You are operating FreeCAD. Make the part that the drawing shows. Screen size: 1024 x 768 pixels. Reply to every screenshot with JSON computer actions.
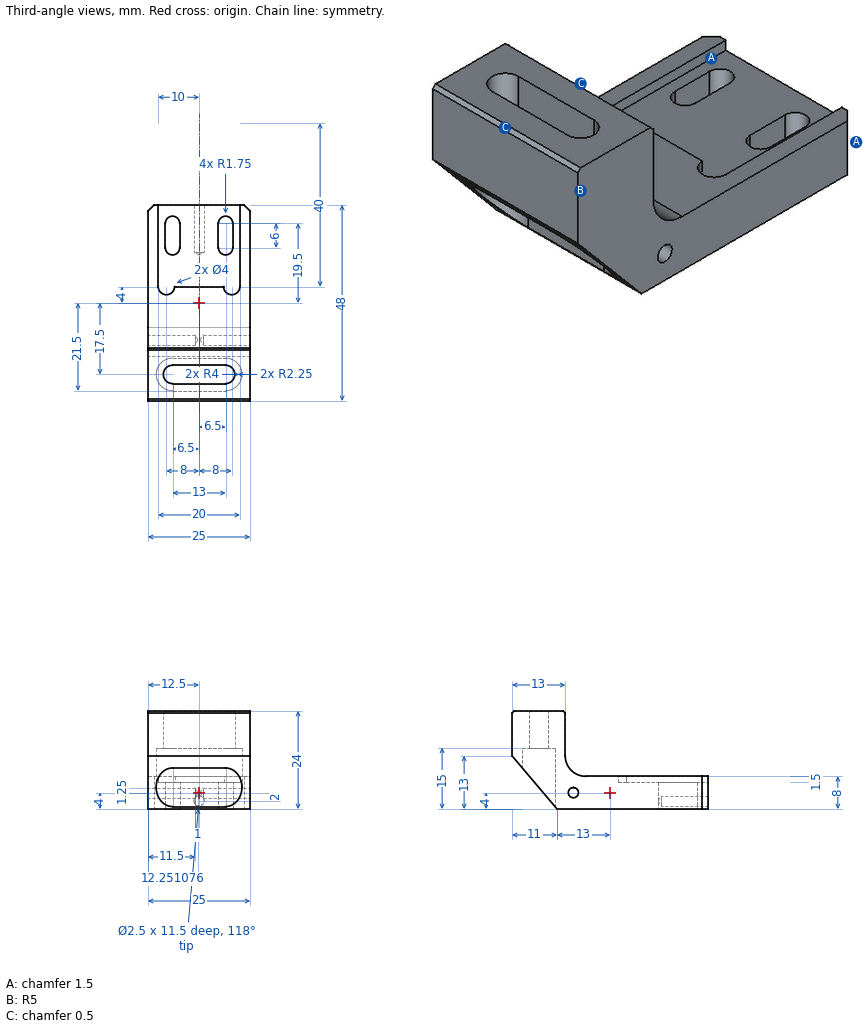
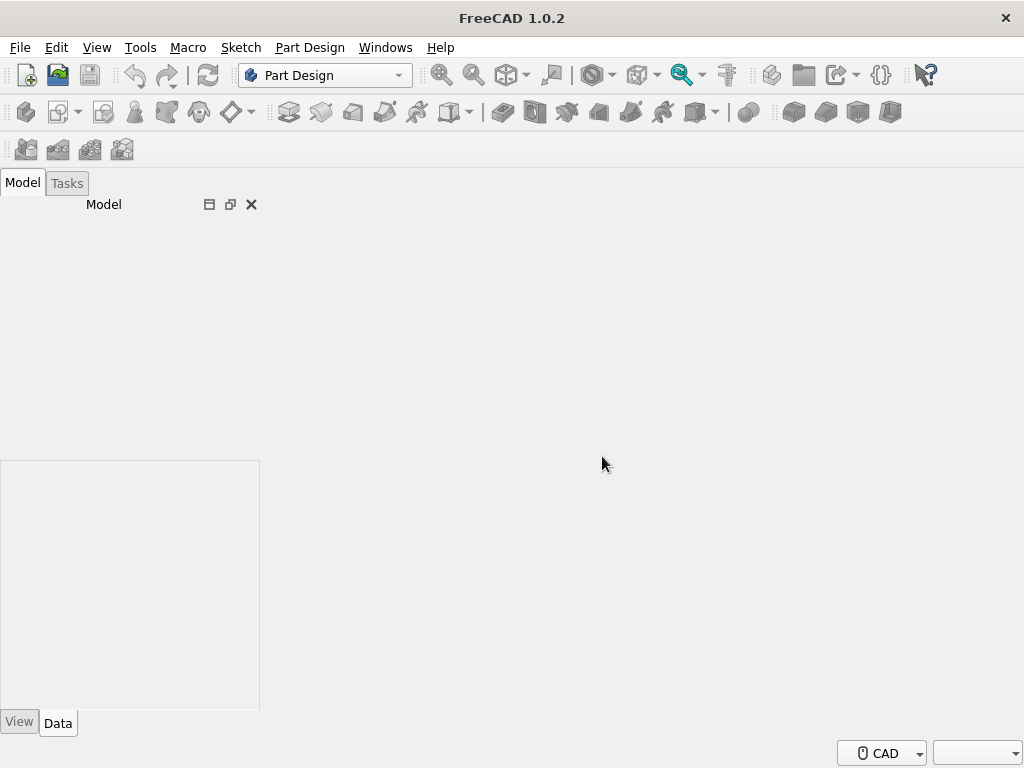
{"action": "left_click", "coordinate": [26, 76]}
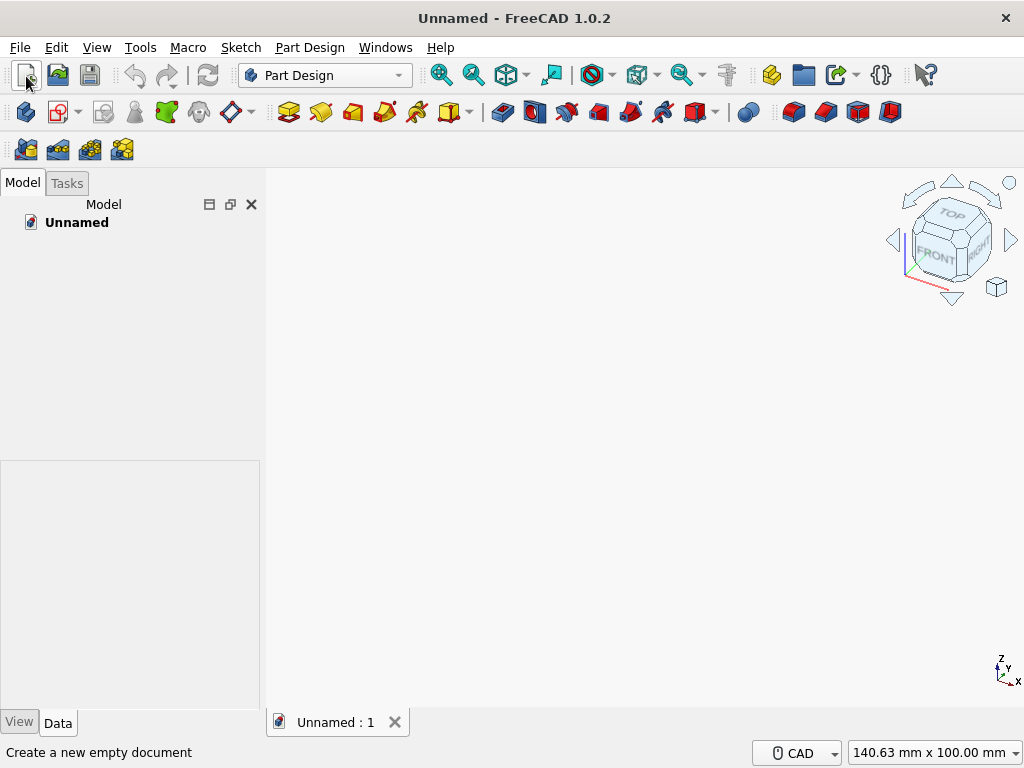
{"action": "left_click", "coordinate": [58, 112]}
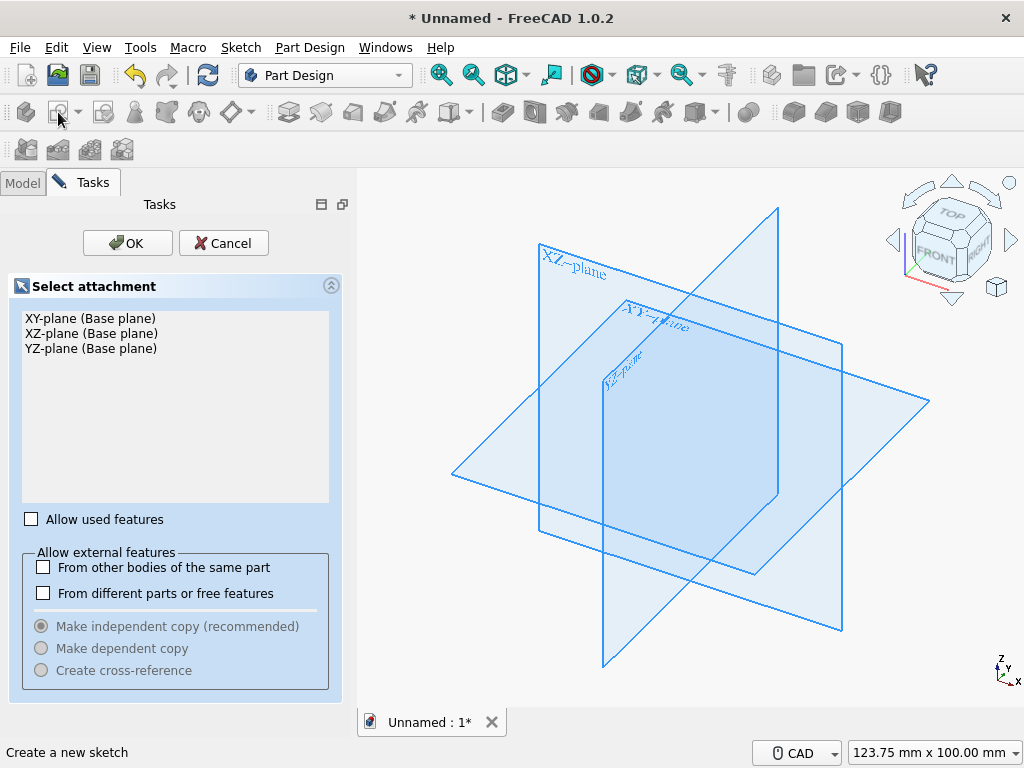
{"action": "left_click", "coordinate": [82, 318]}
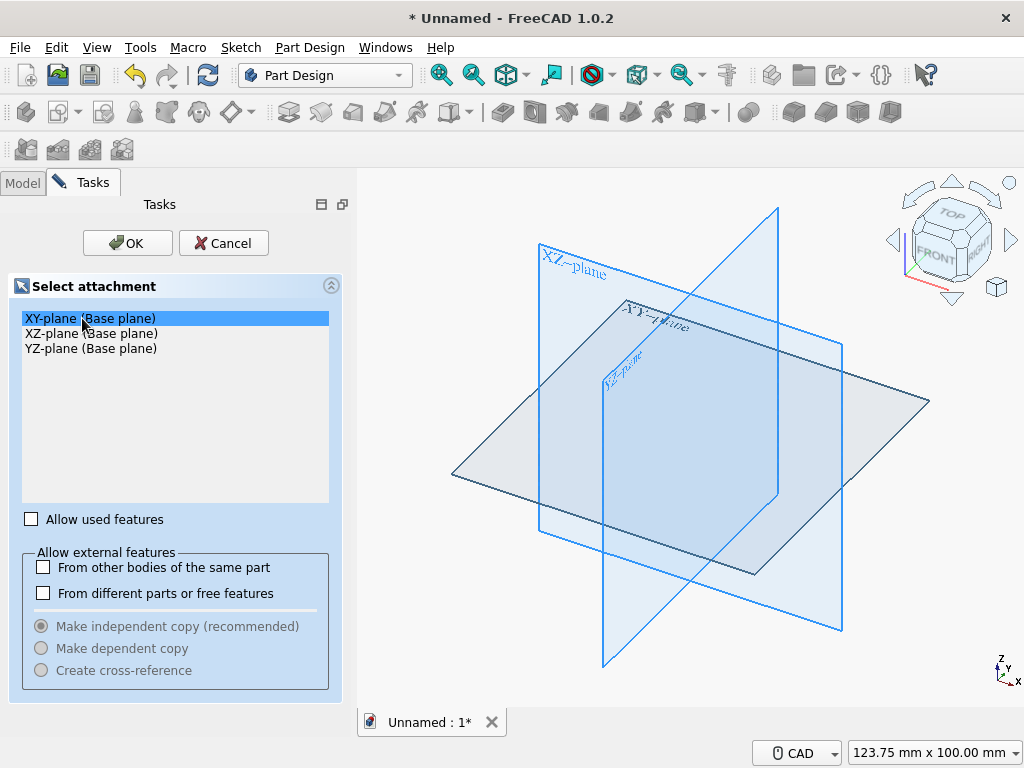
{"action": "left_click", "coordinate": [128, 243]}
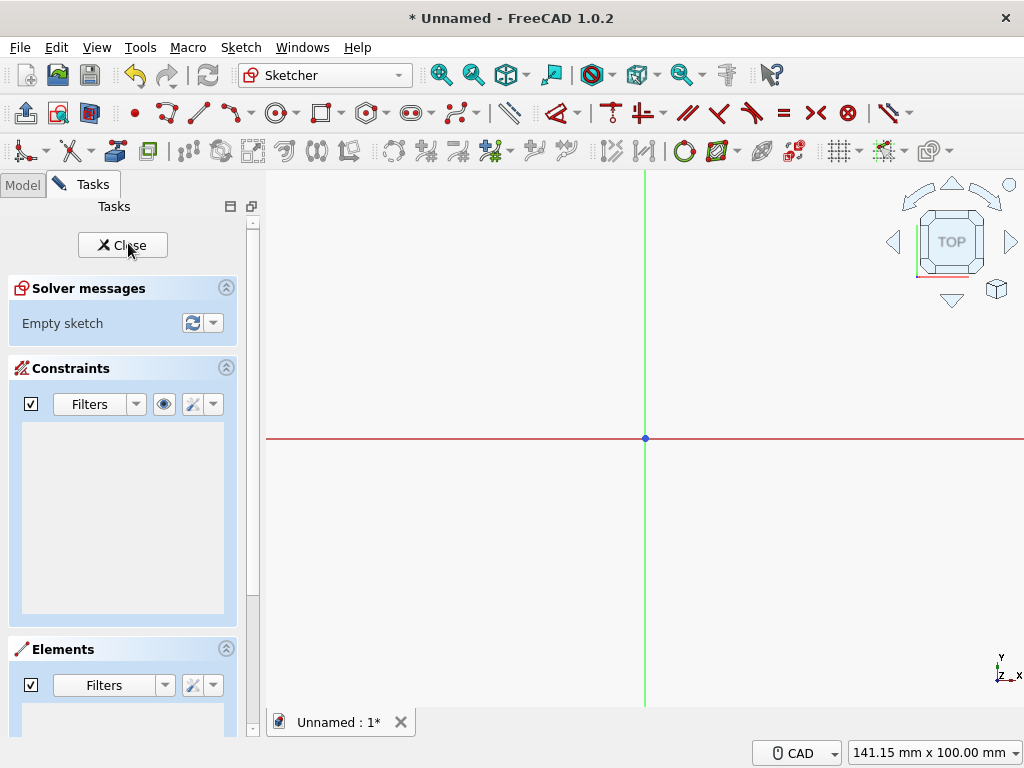
{"action": "left_click", "coordinate": [344, 114]}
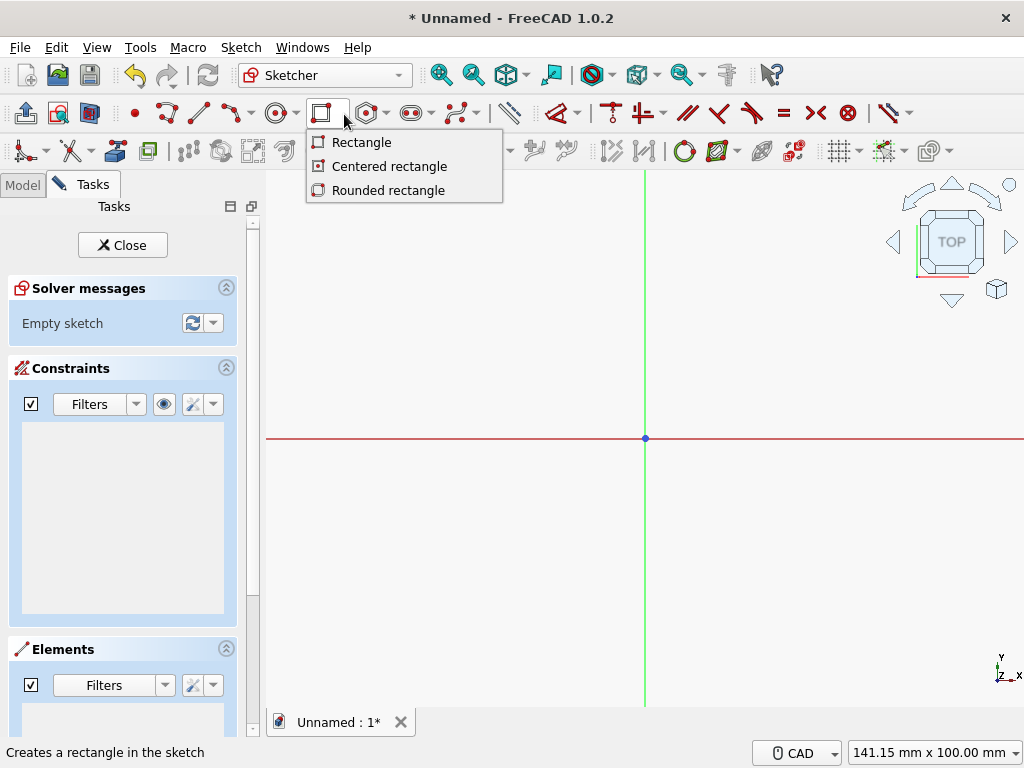
{"action": "left_click", "coordinate": [404, 166]}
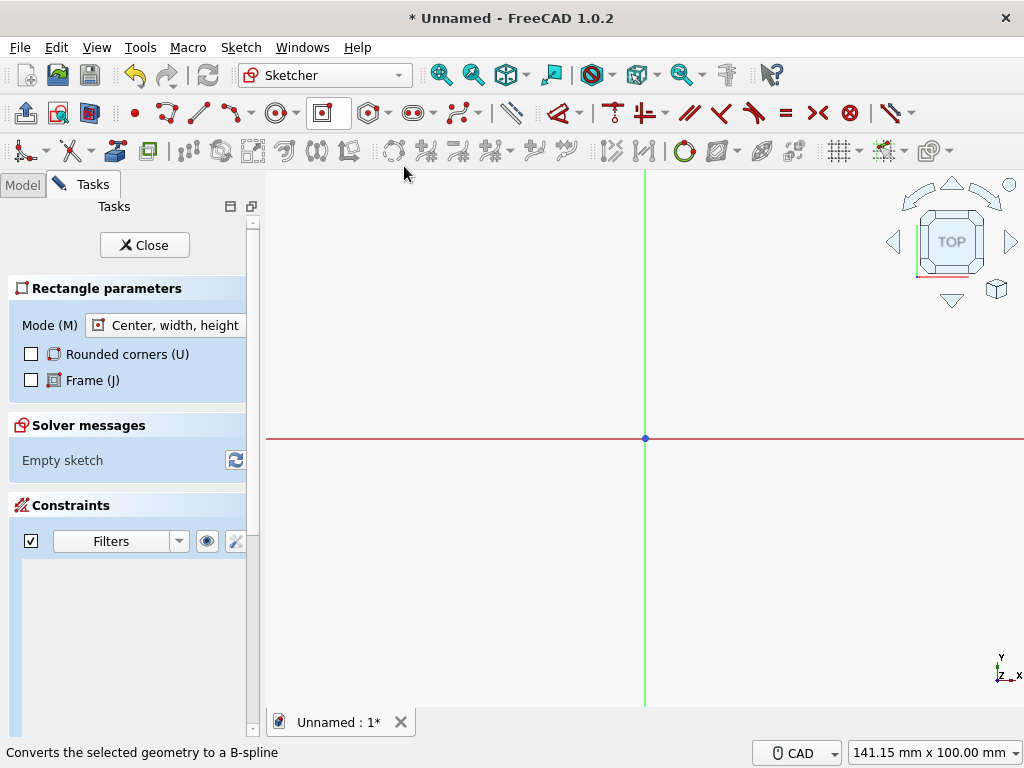
{"action": "left_click", "coordinate": [645, 438]}
{"action": "mouse_move", "coordinate": [712, 310]}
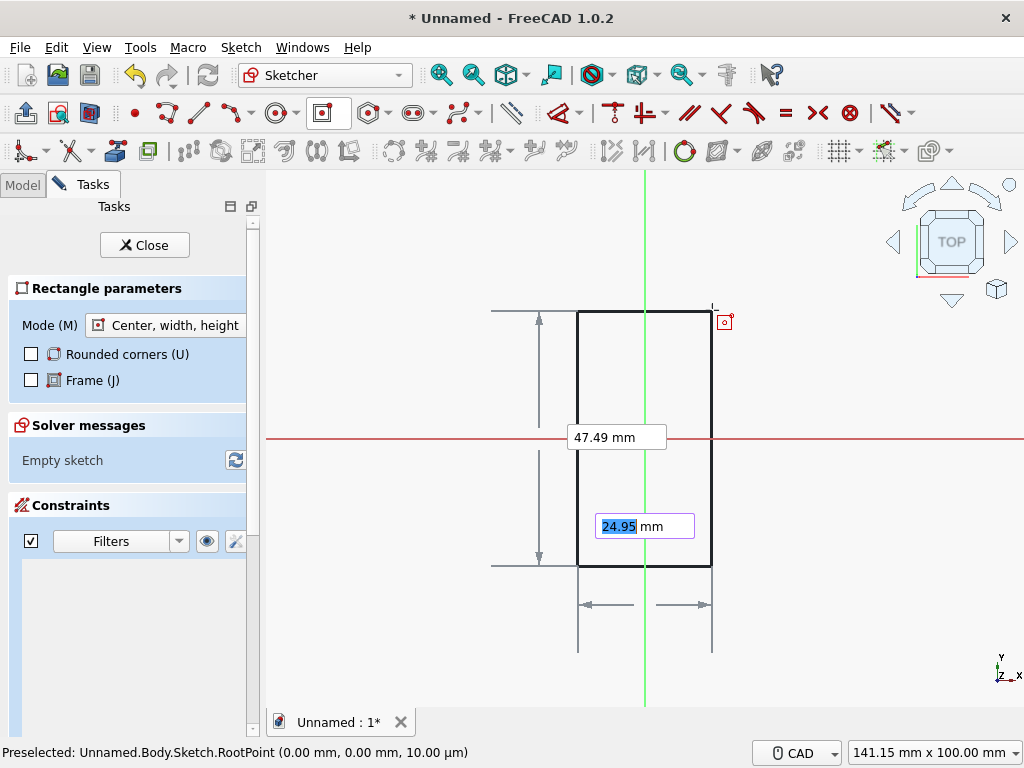
{"action": "type", "text": "25"}
{"action": "key", "text": "Tab"}
{"action": "type", "text": "48"}
{"action": "key", "text": "Return"}
{"action": "key", "text": "Escape"}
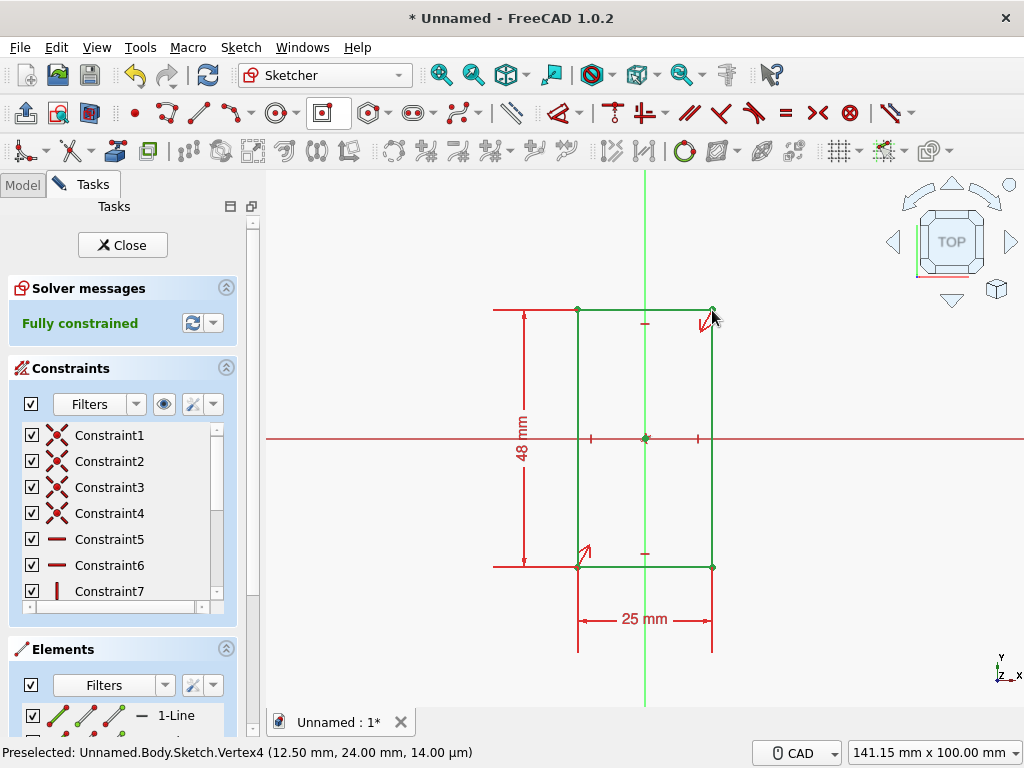
{"action": "left_click", "coordinate": [123, 245]}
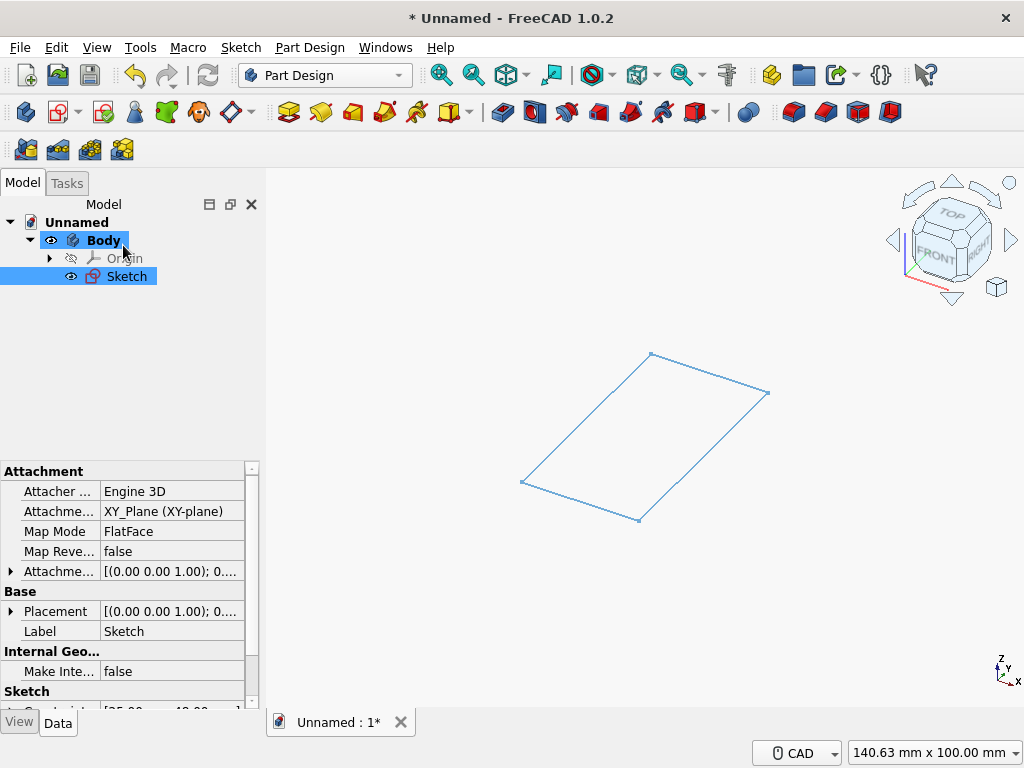
{"action": "left_click", "coordinate": [290, 112]}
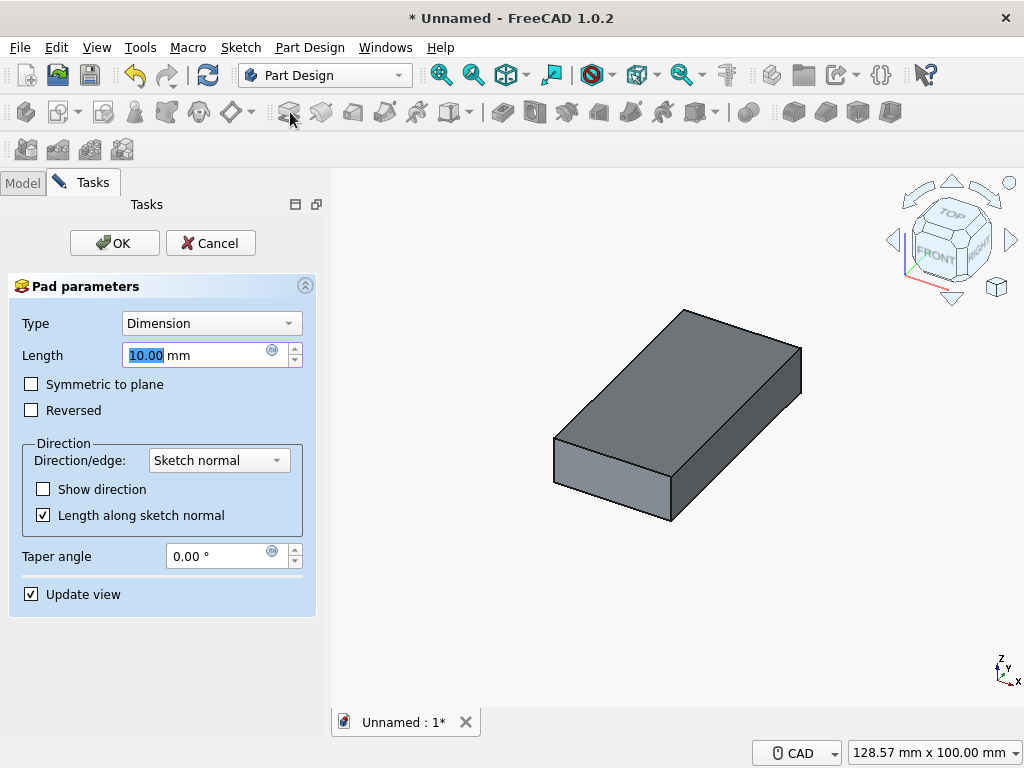
{"action": "type", "text": "8"}
{"action": "key", "text": "Tab"}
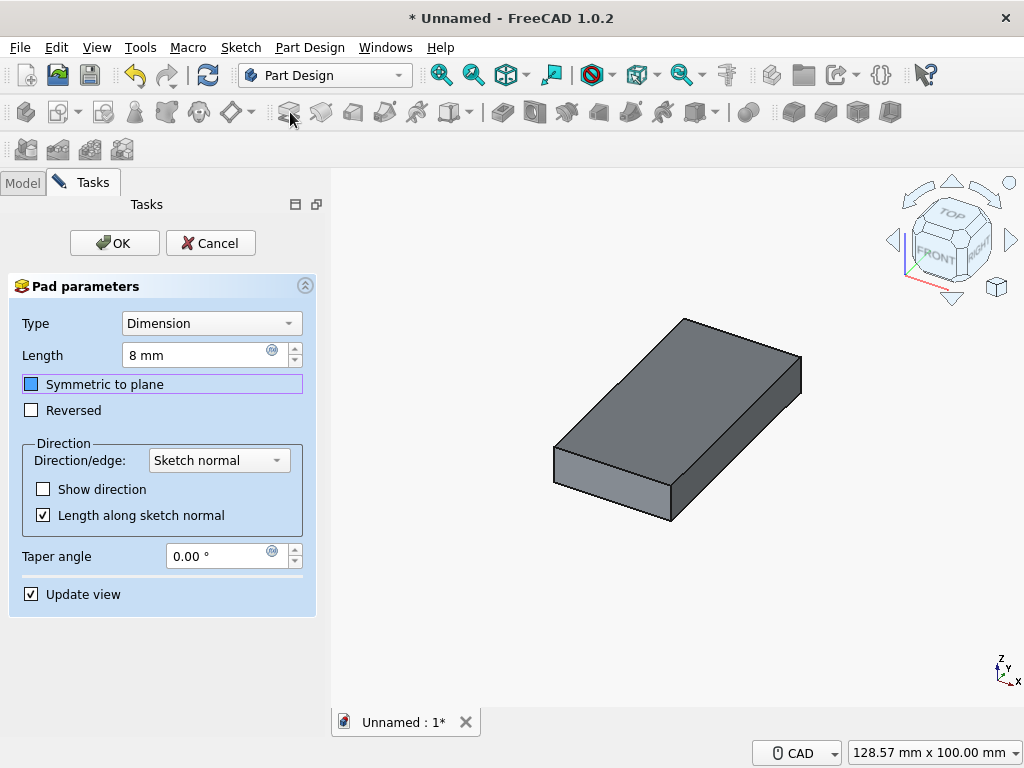
{"action": "left_click", "coordinate": [30, 384]}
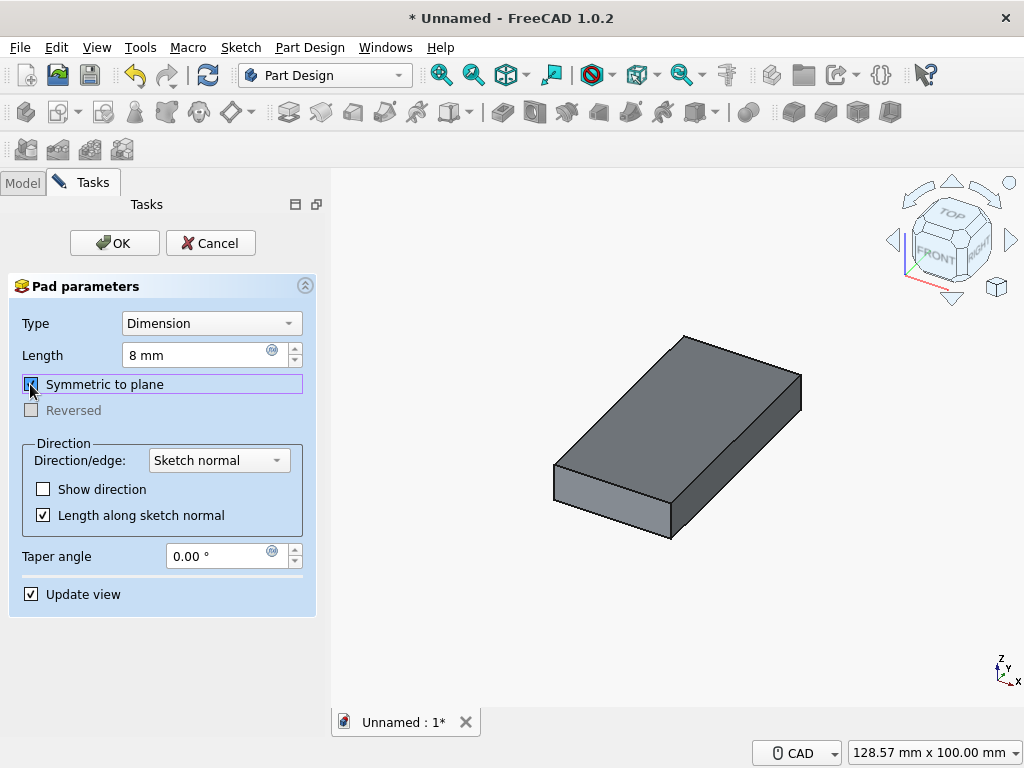
{"action": "left_click", "coordinate": [115, 243]}